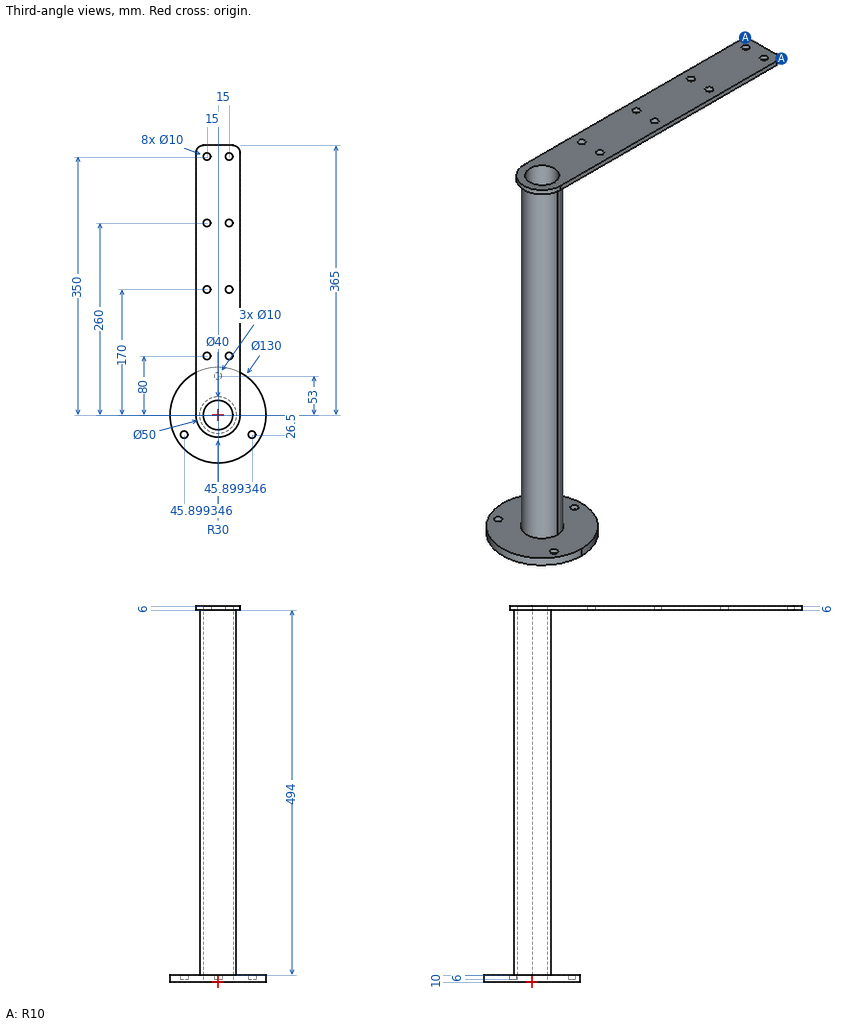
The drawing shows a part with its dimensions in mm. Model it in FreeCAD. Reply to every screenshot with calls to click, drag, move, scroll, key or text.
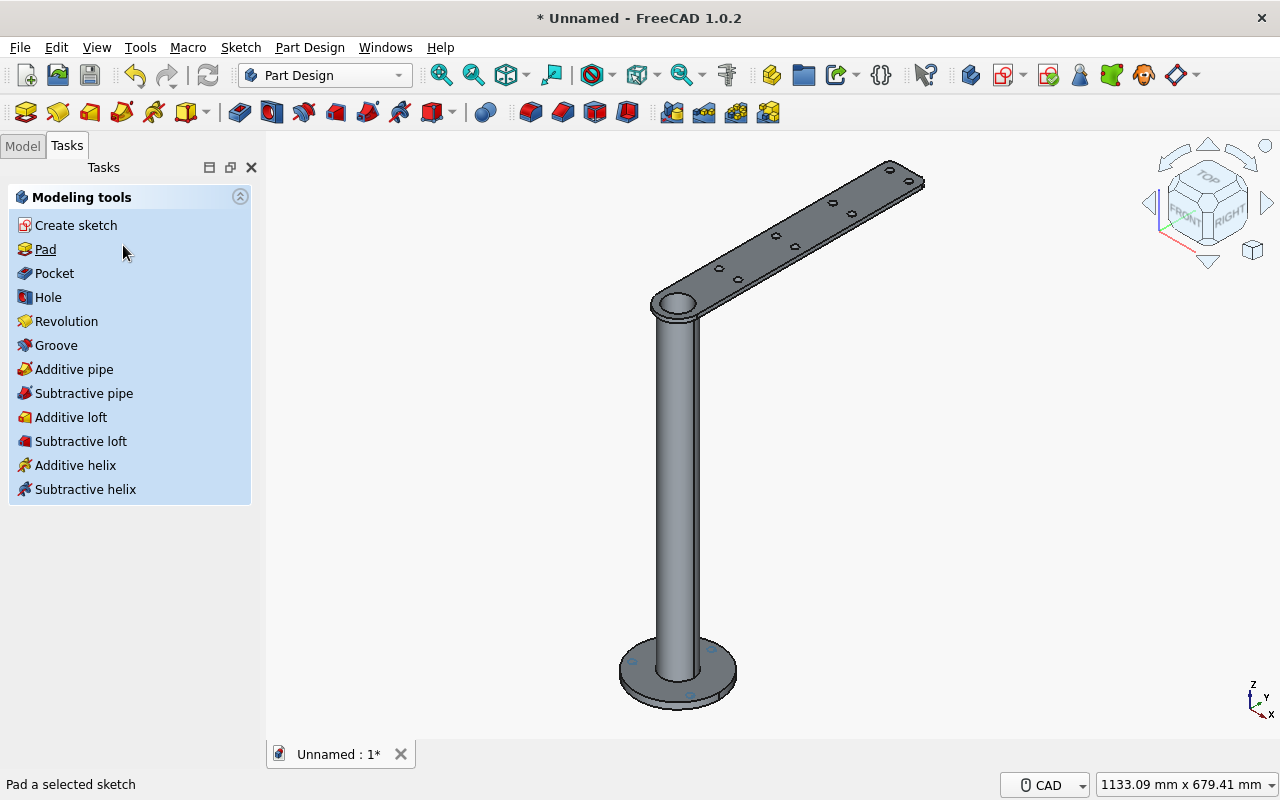
click(240, 112)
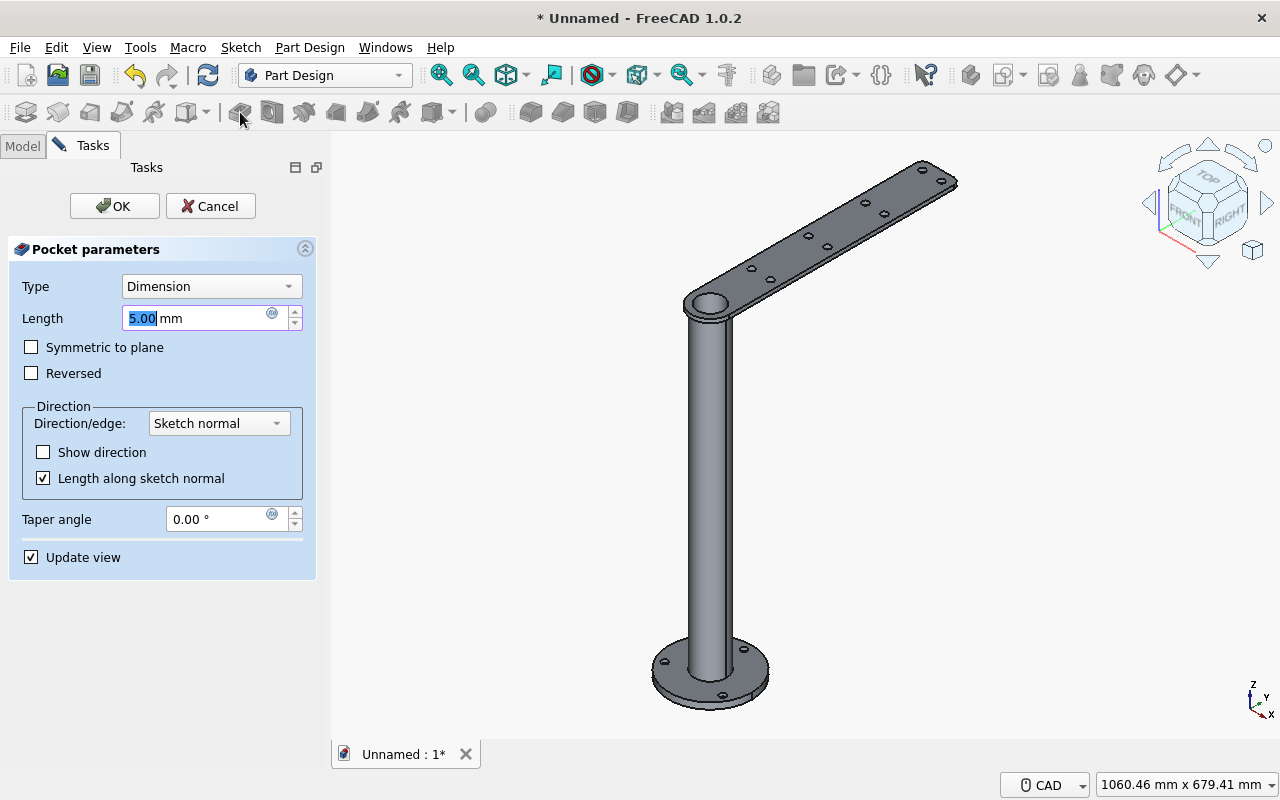
text(6)
key(Tab)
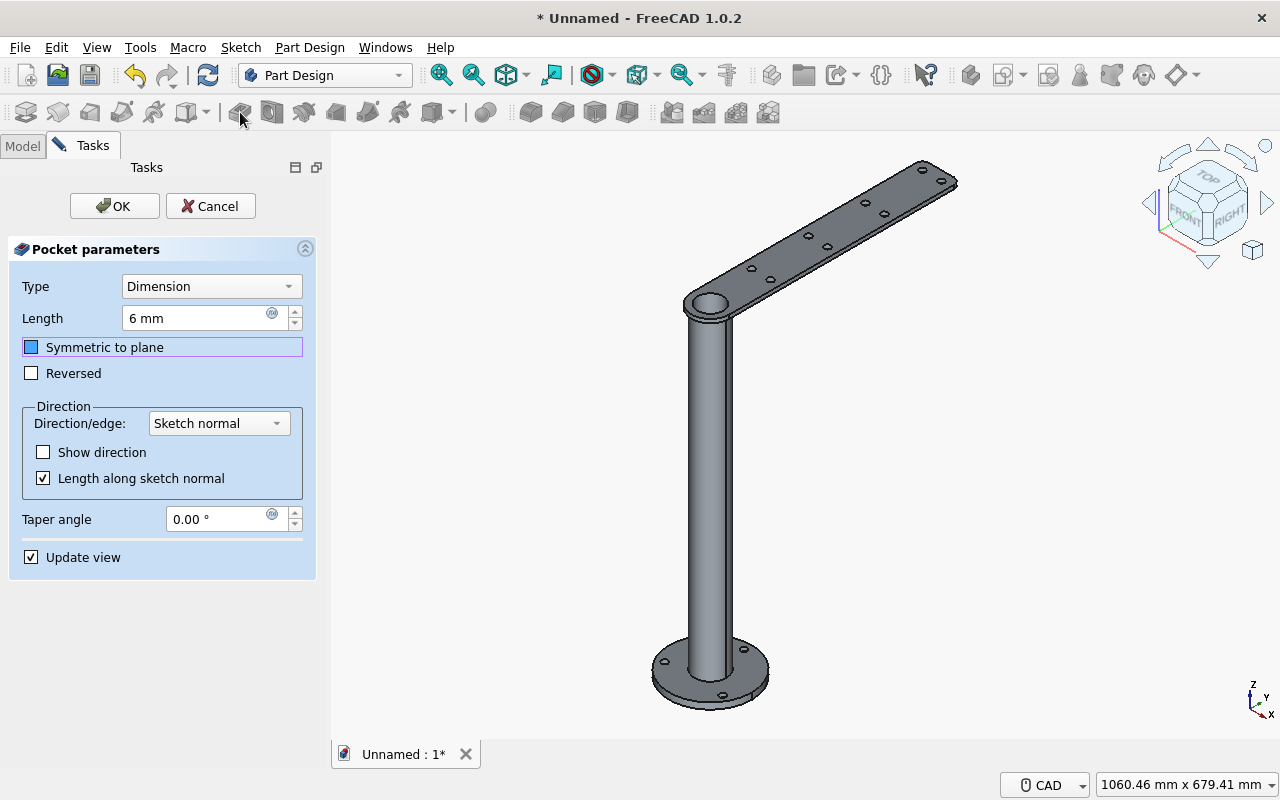
click(115, 206)